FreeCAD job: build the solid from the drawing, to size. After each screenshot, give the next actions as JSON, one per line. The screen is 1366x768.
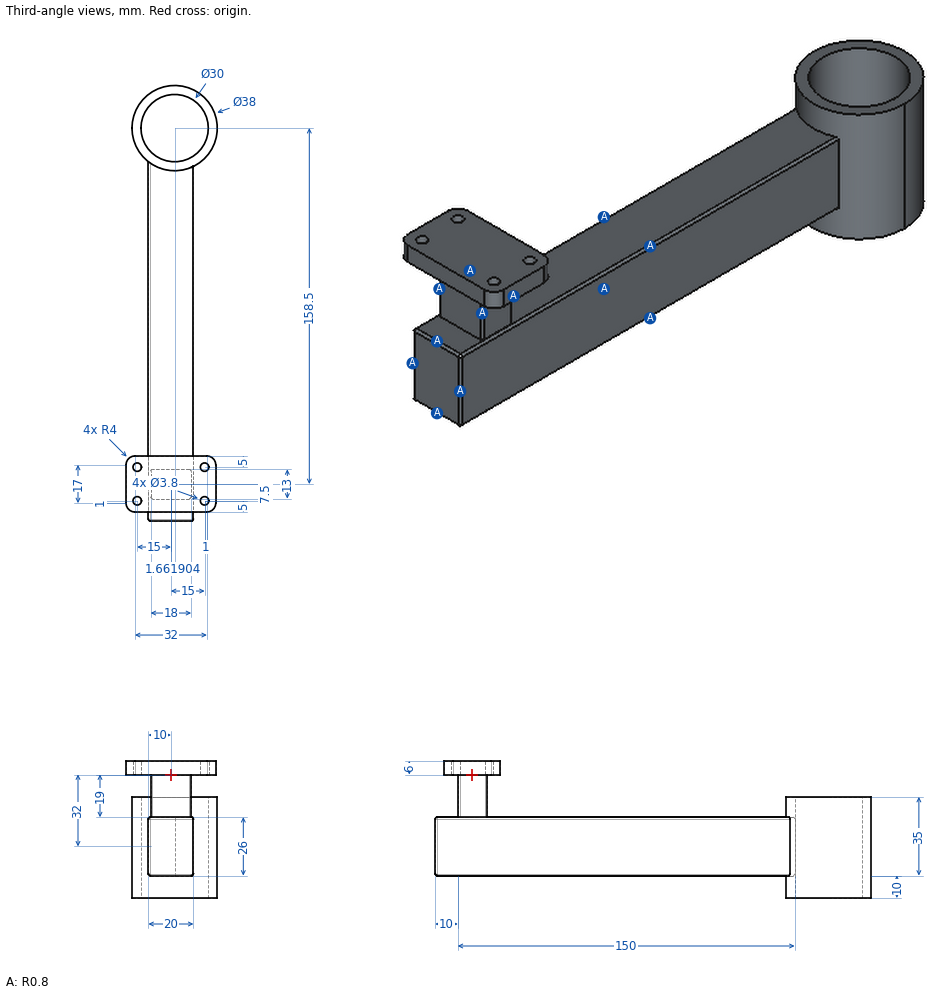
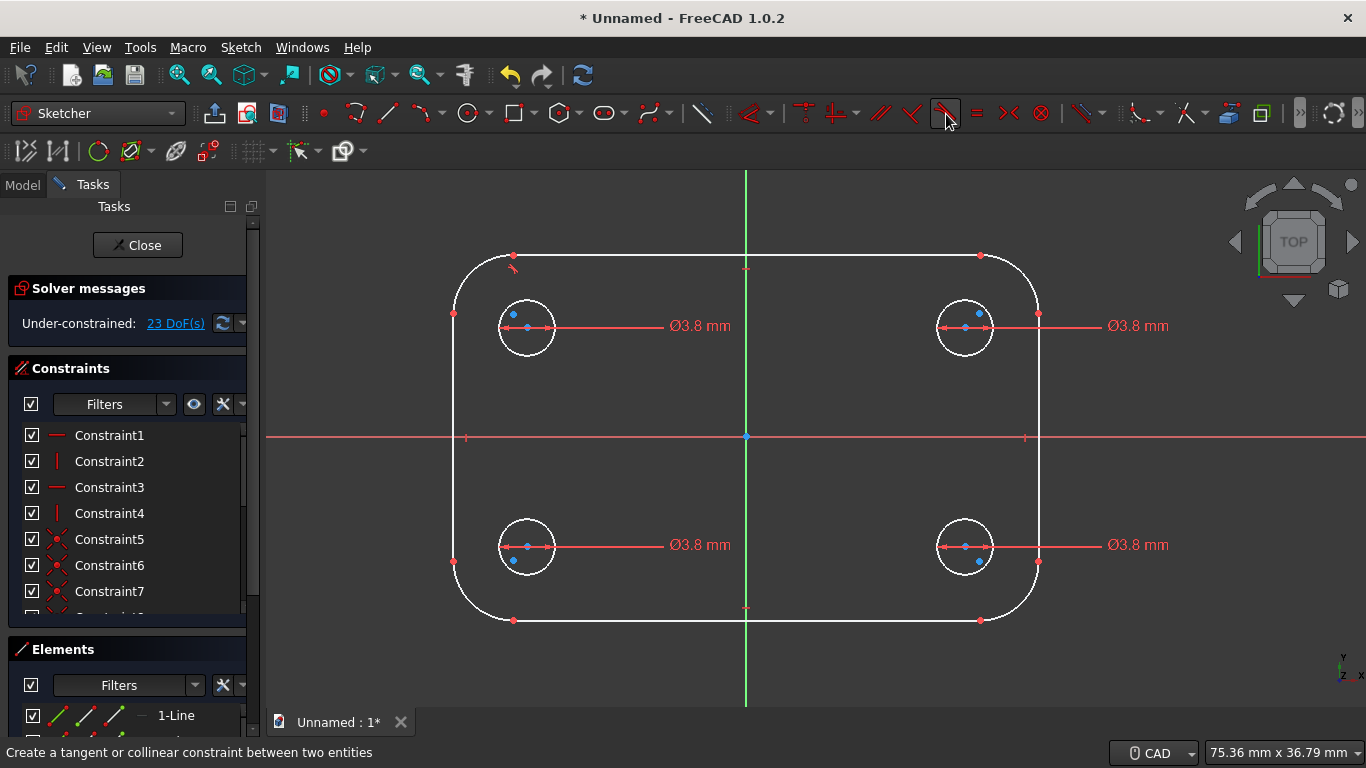
{"action": "left_click", "coordinate": [840, 255]}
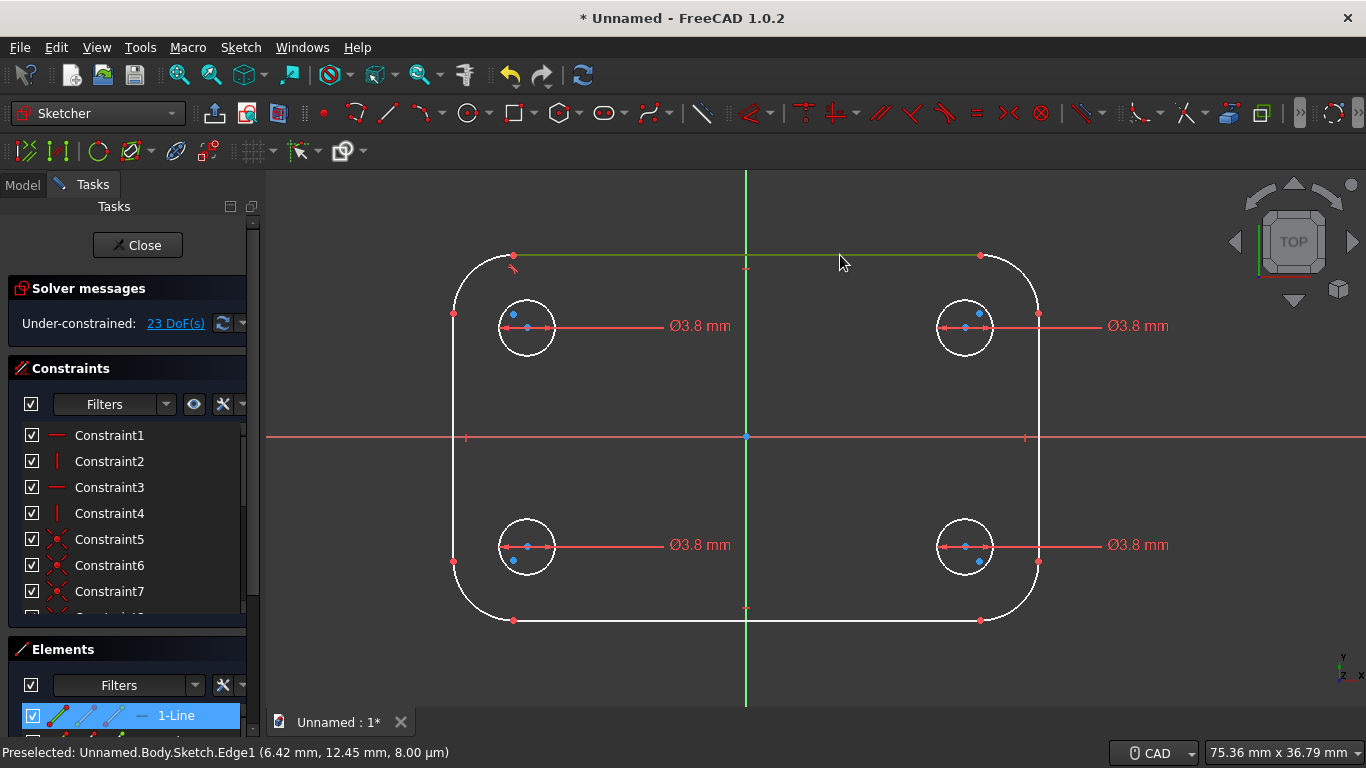
{"action": "left_click", "coordinate": [1032, 287]}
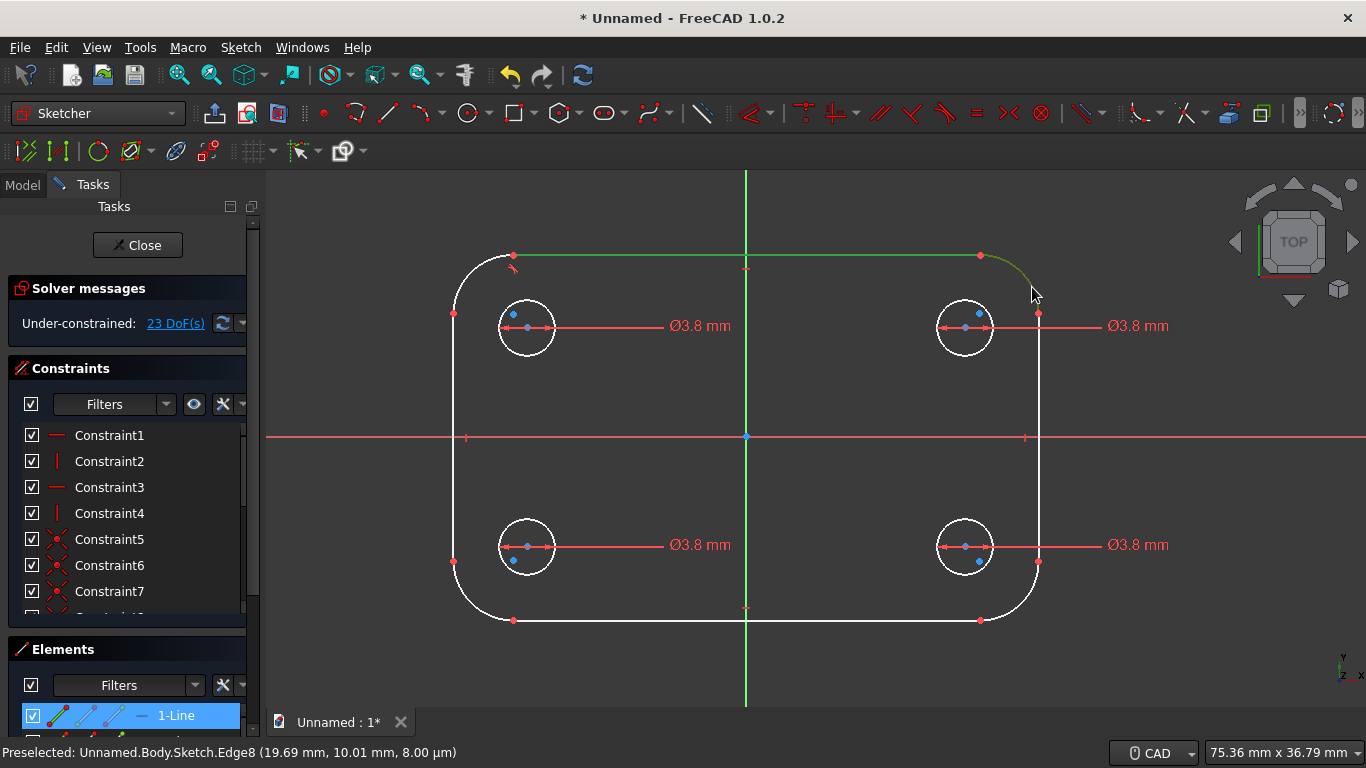
{"action": "left_click", "coordinate": [946, 114]}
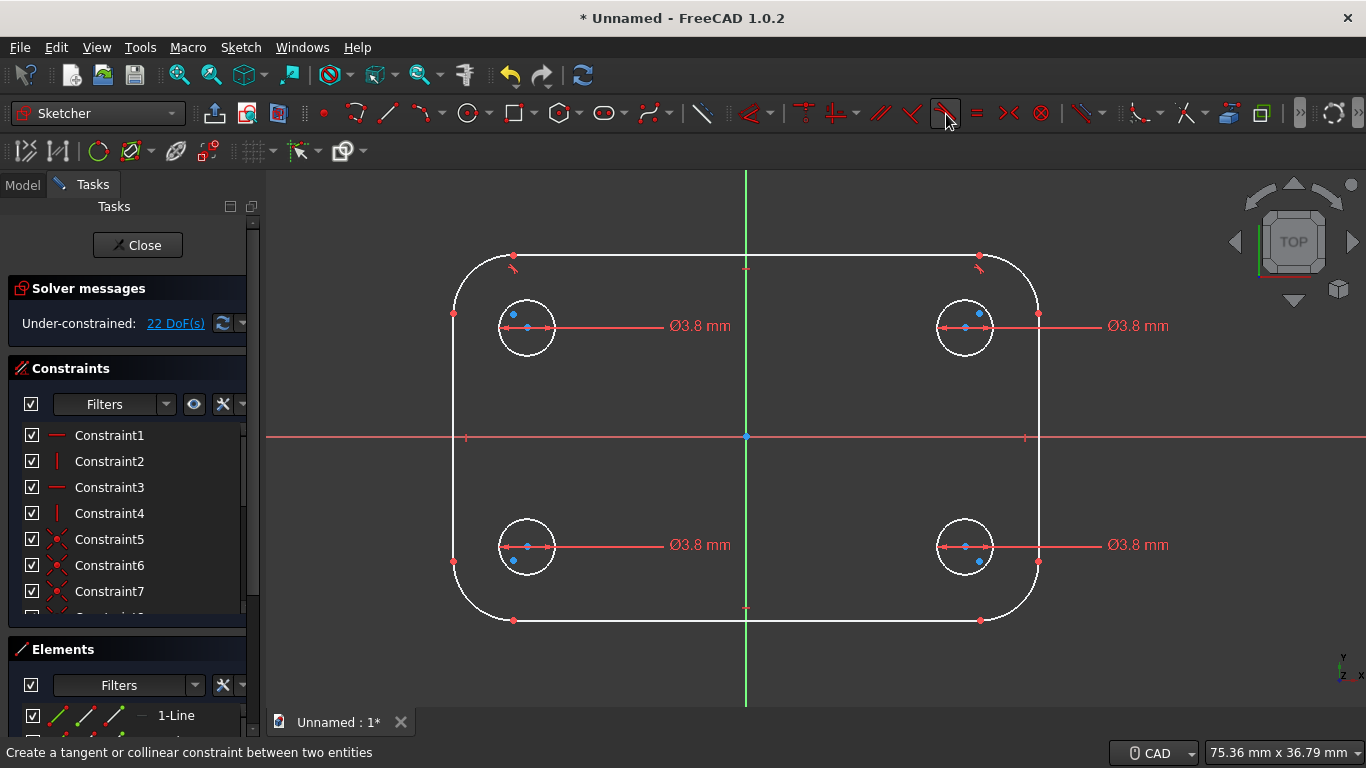
{"action": "left_click", "coordinate": [453, 388]}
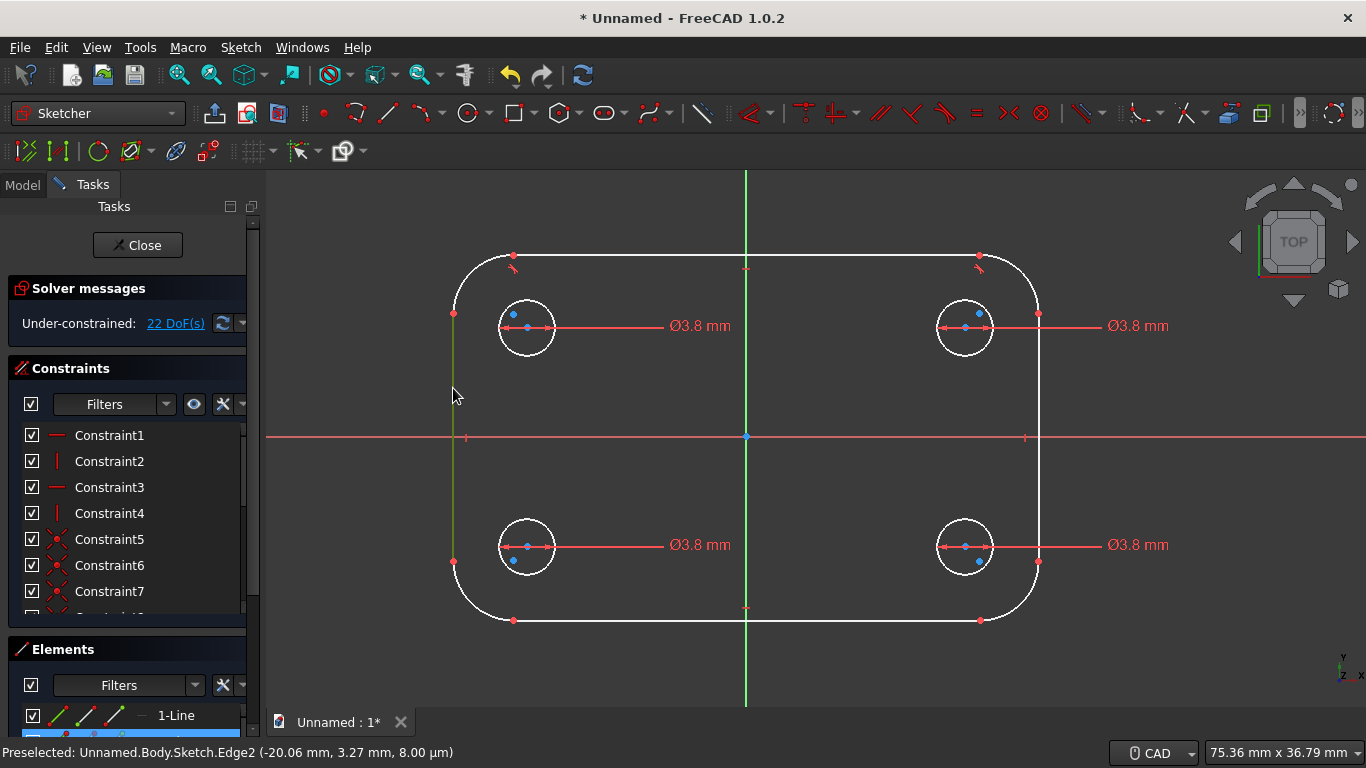
{"action": "left_click", "coordinate": [486, 261]}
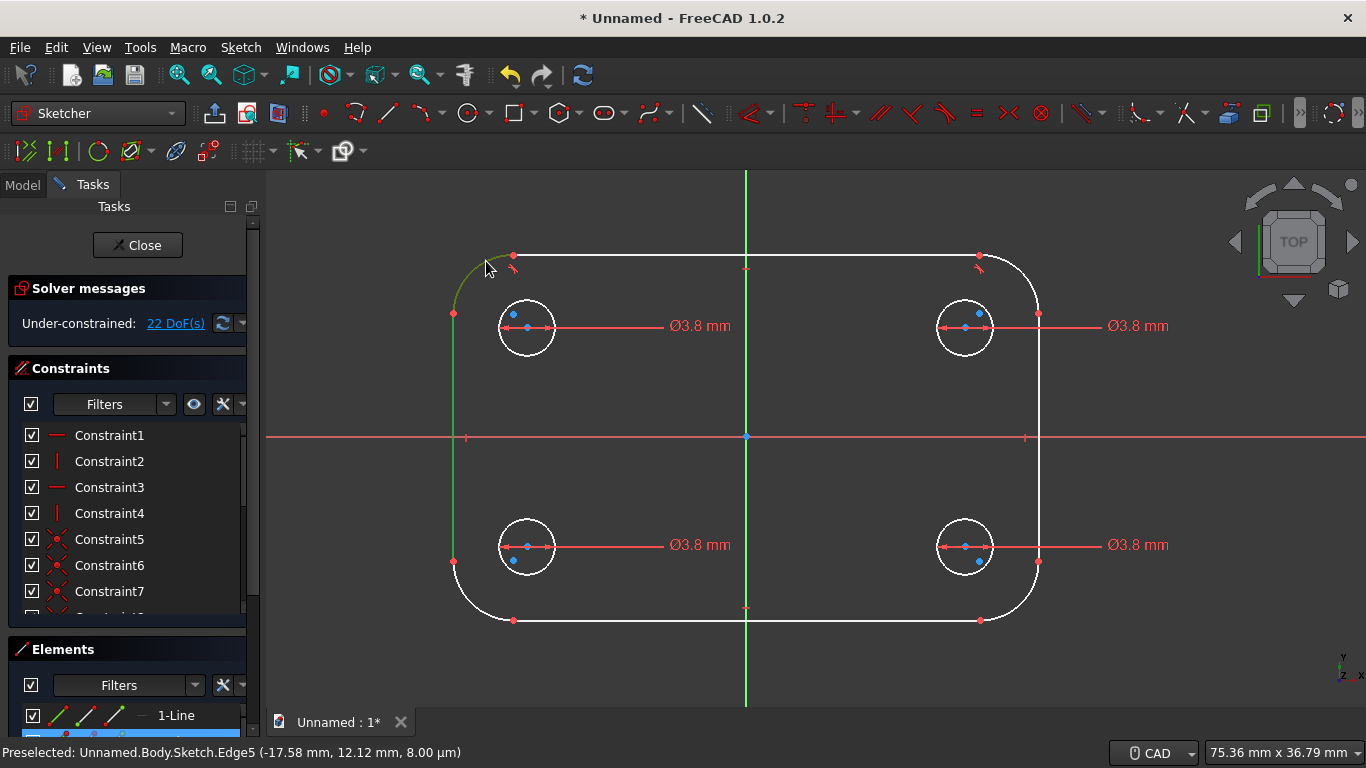
{"action": "left_click", "coordinate": [946, 114]}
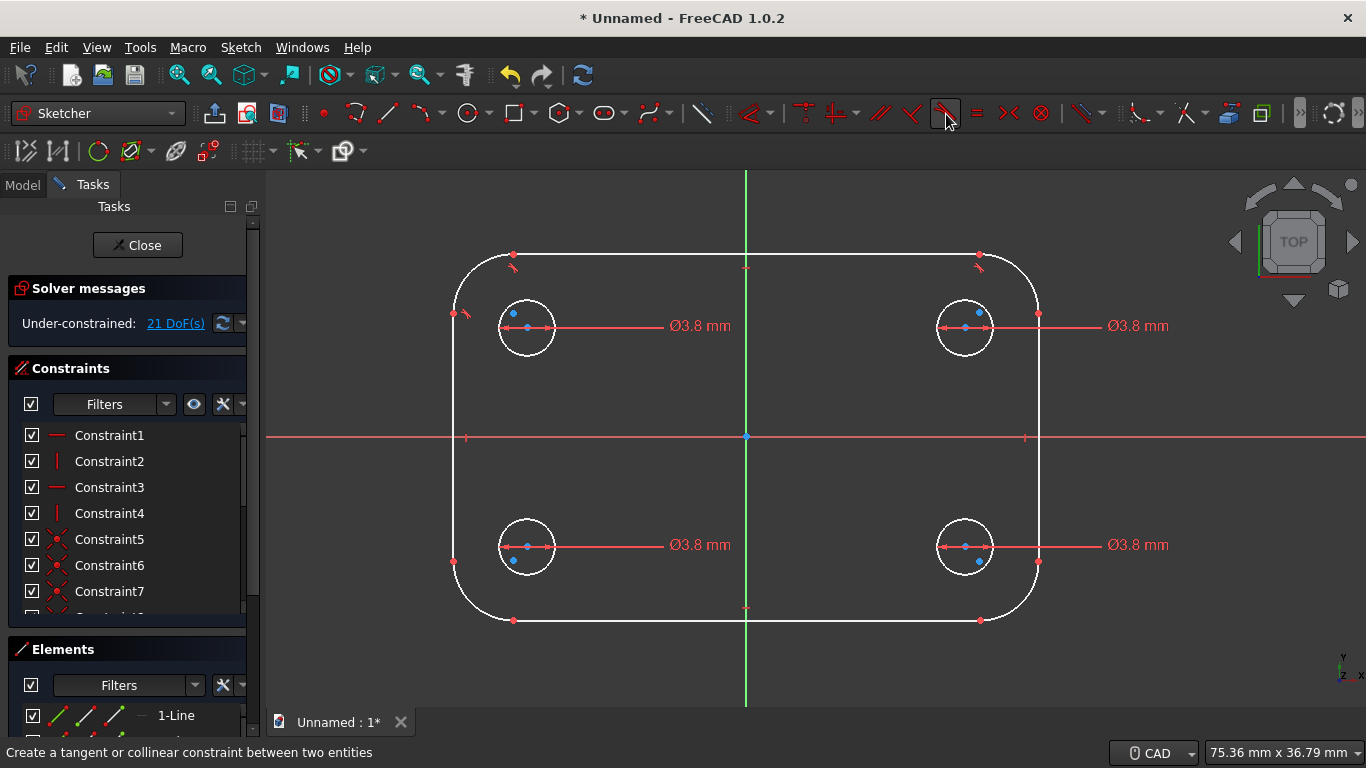
{"action": "left_click", "coordinate": [453, 388]}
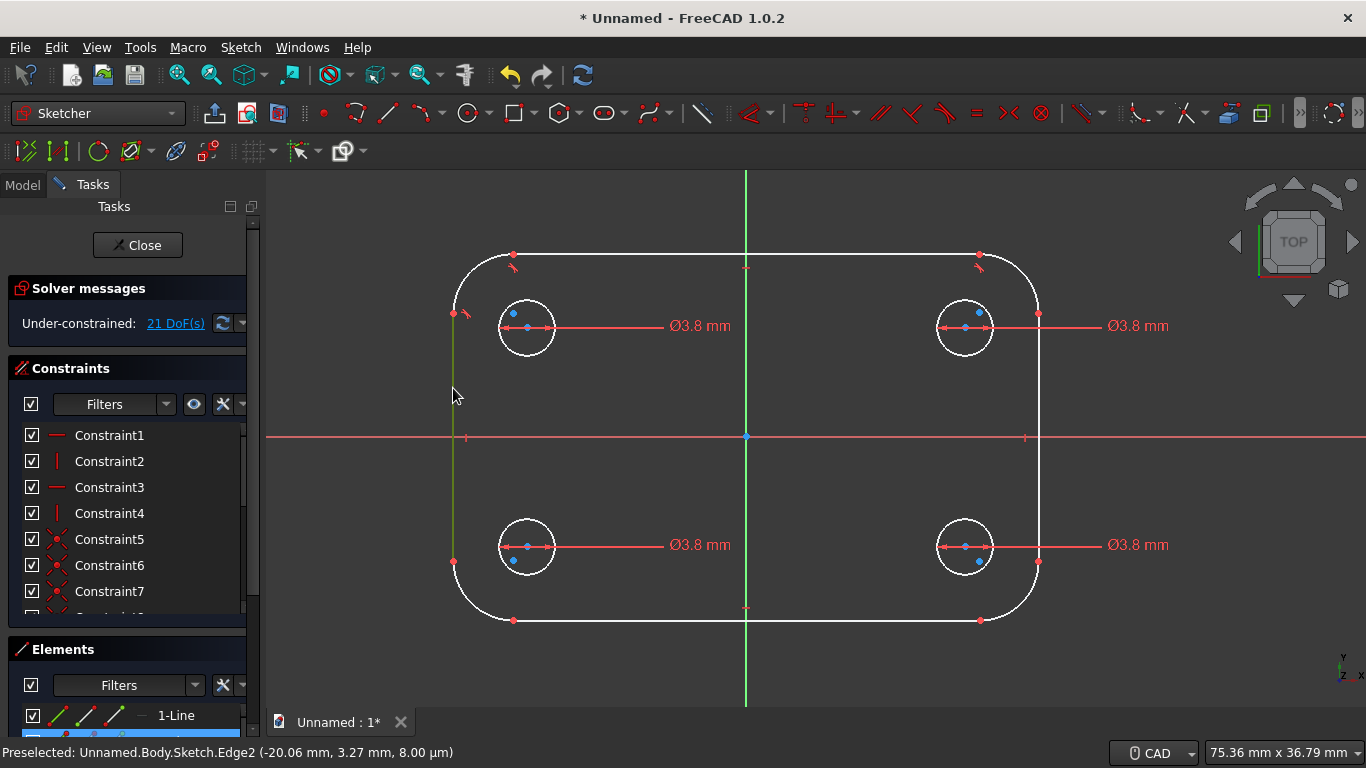
{"action": "left_click", "coordinate": [461, 588]}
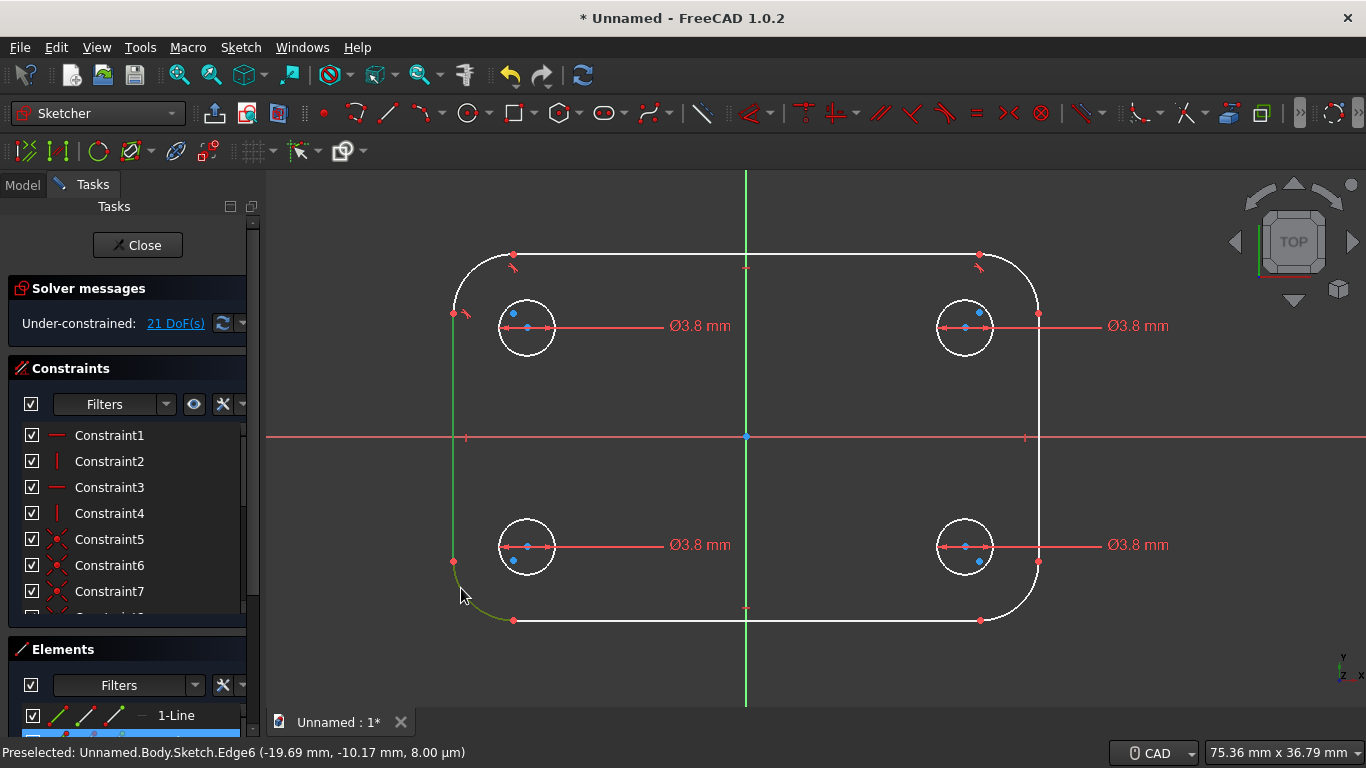
{"action": "left_click", "coordinate": [946, 114]}